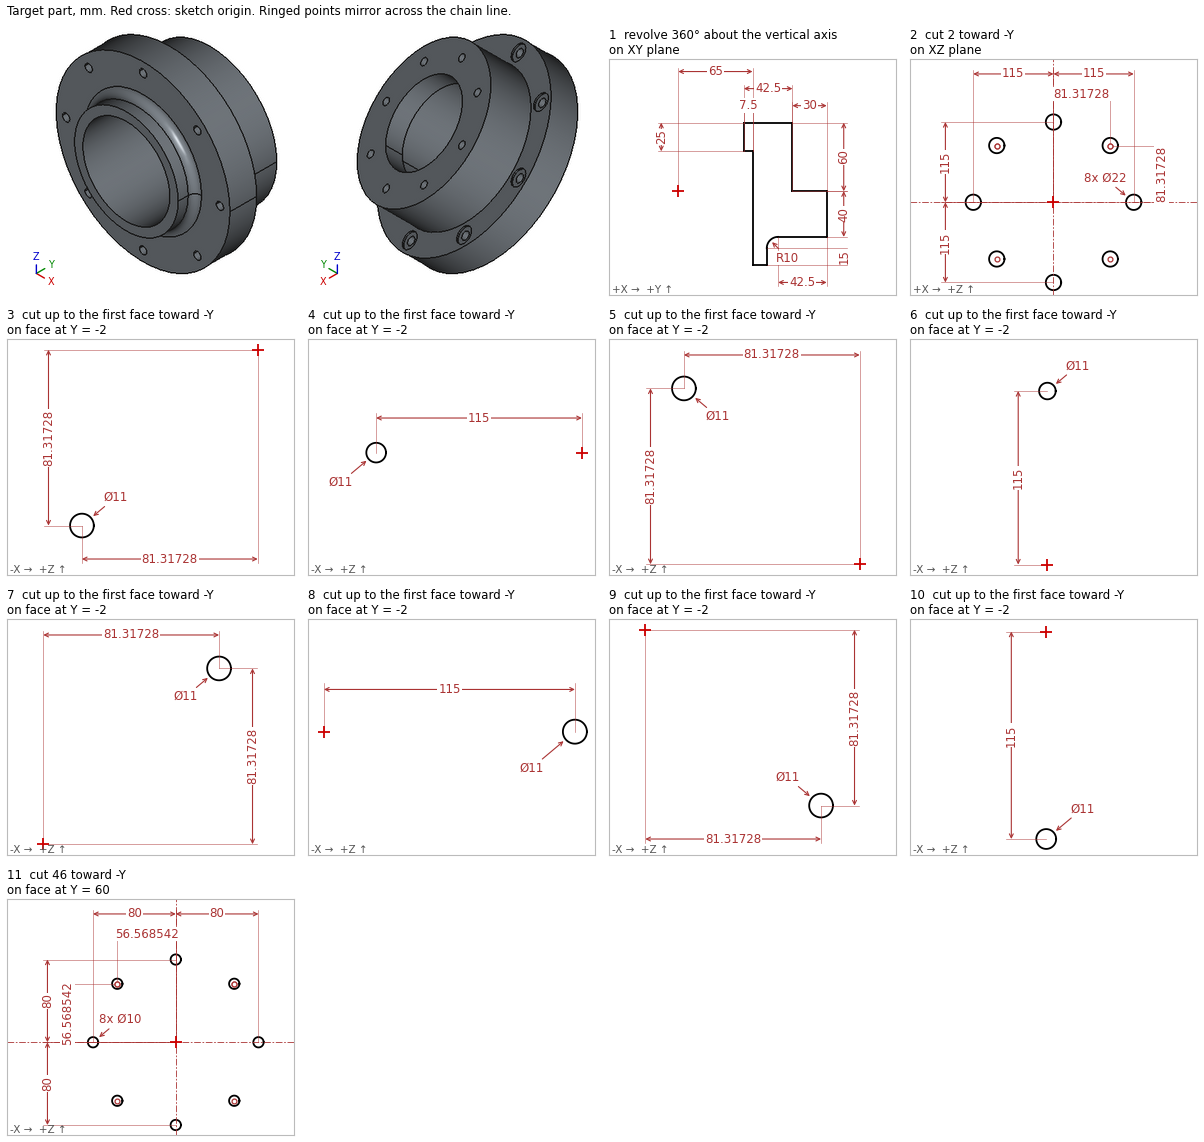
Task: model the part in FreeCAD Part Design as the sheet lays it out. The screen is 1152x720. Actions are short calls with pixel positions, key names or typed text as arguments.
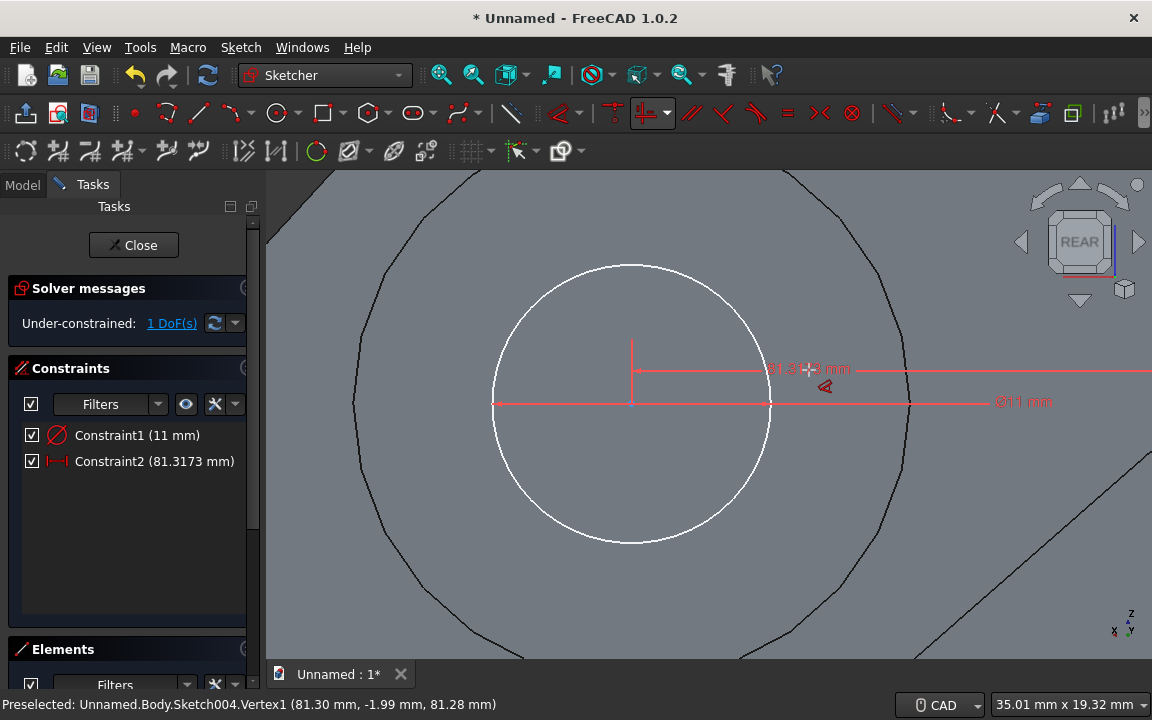
click(632, 404)
click(598, 518)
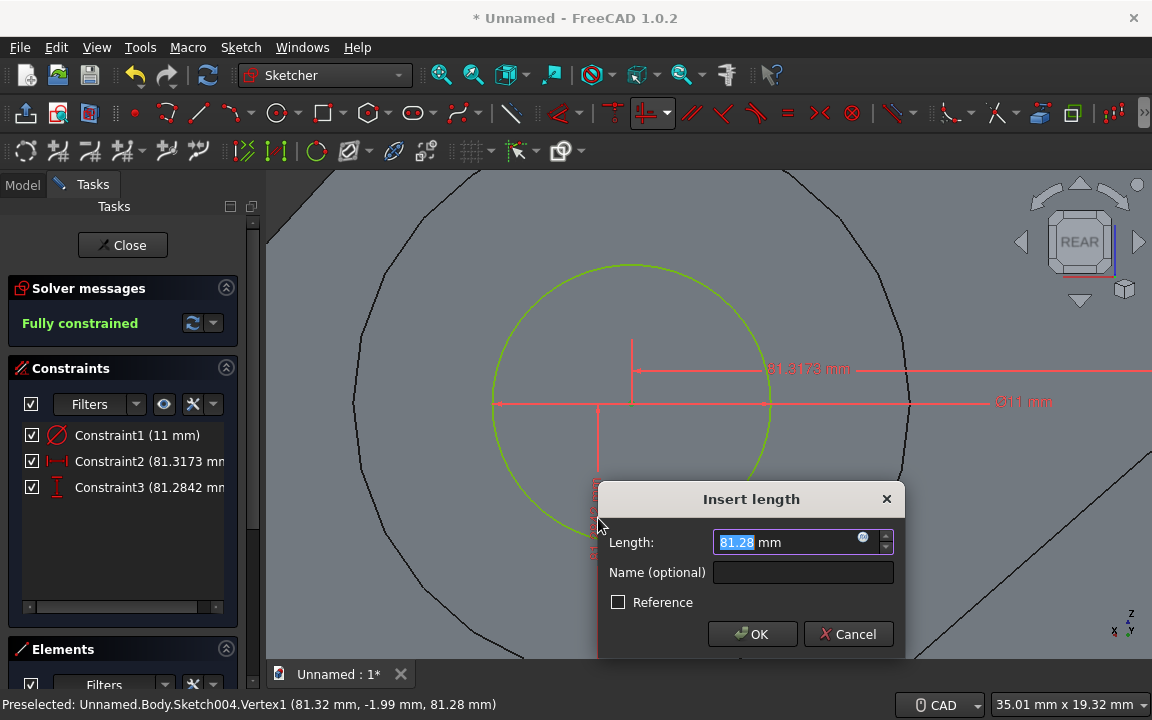
text(81.31728)
key(Return)
key(Escape)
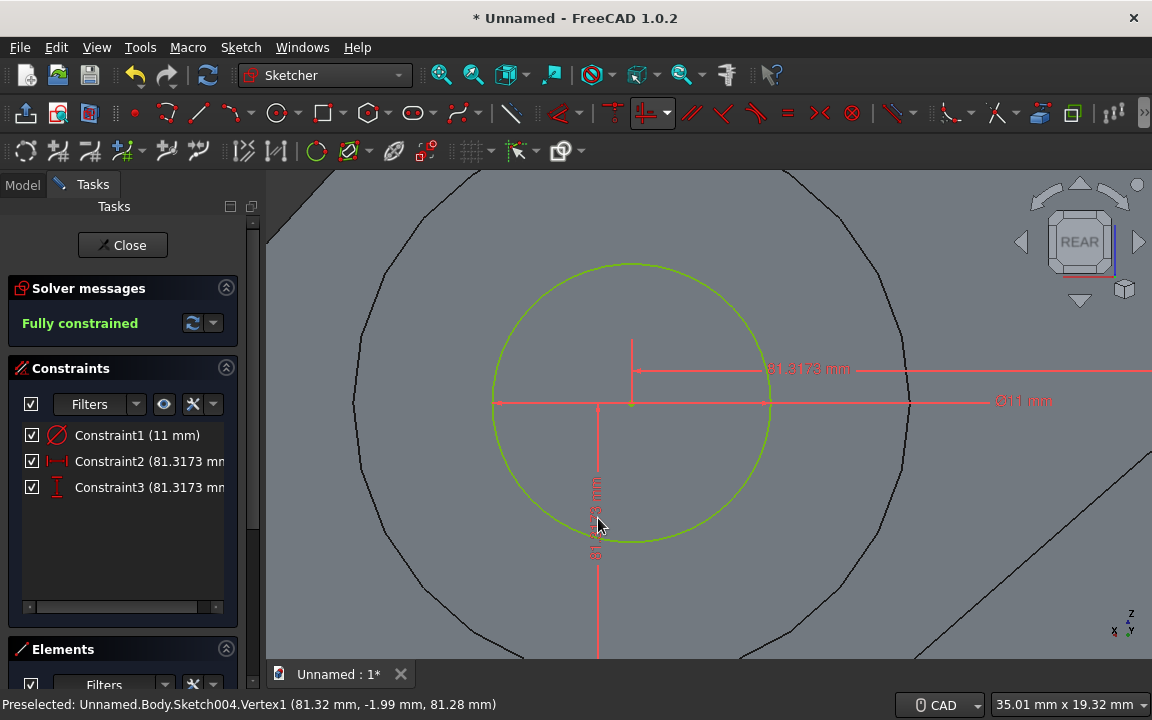
click(123, 245)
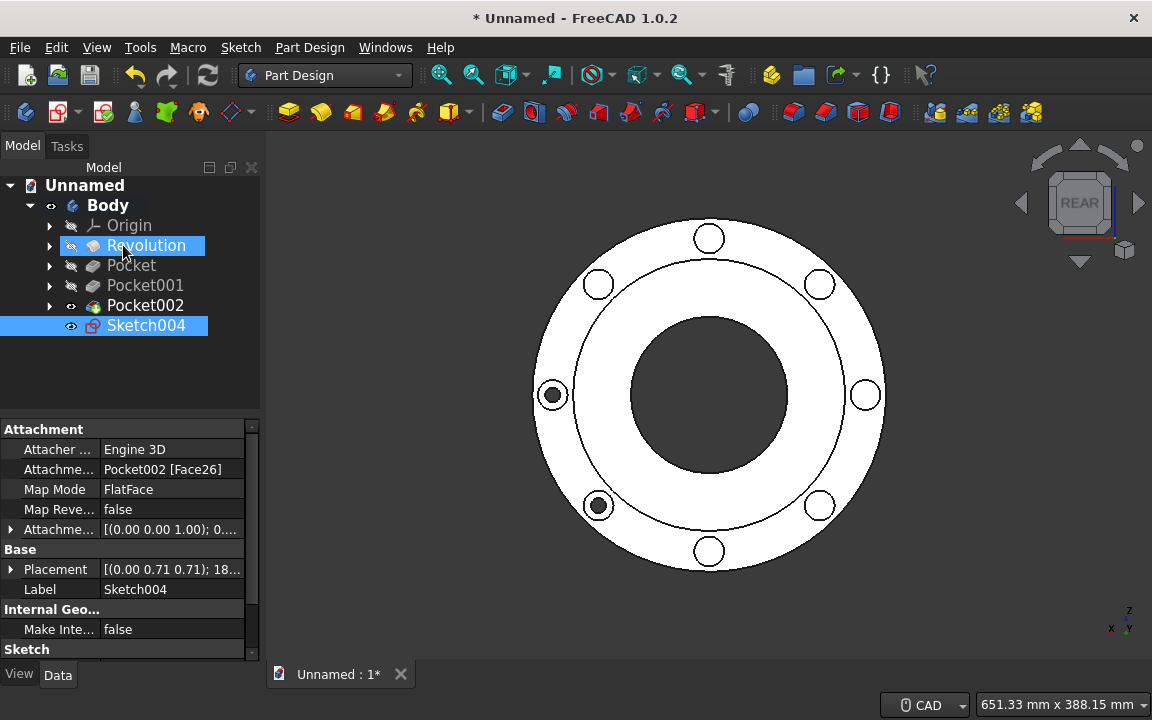
click(504, 112)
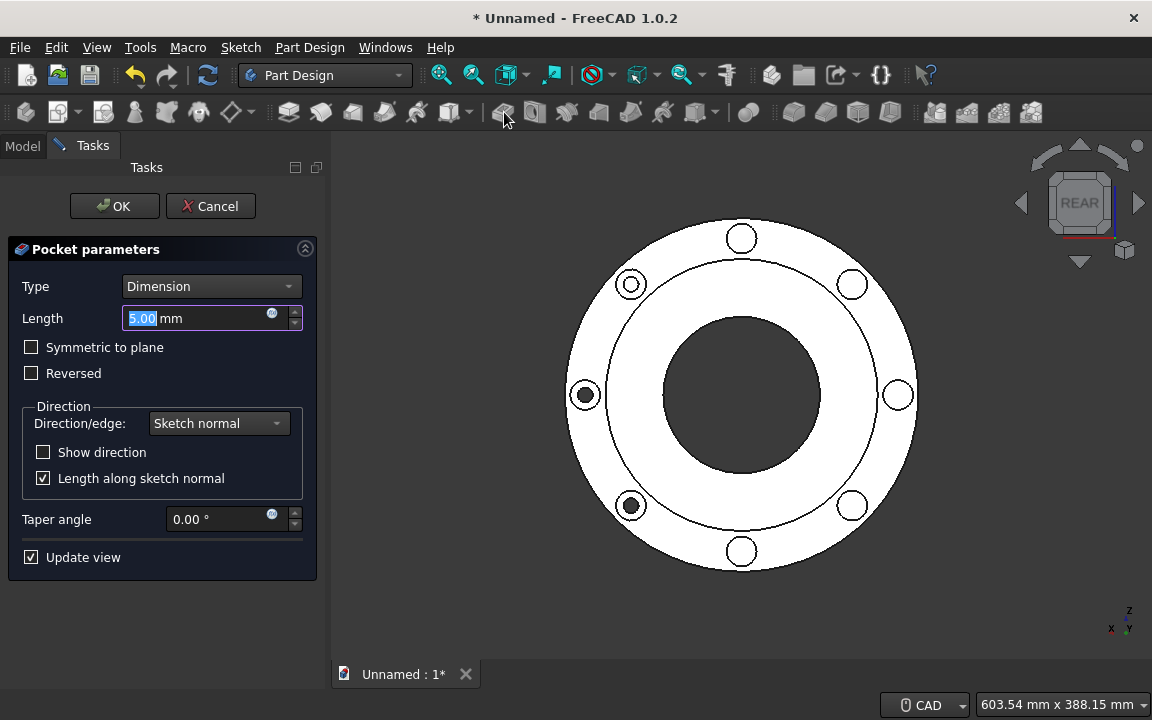
click(212, 286)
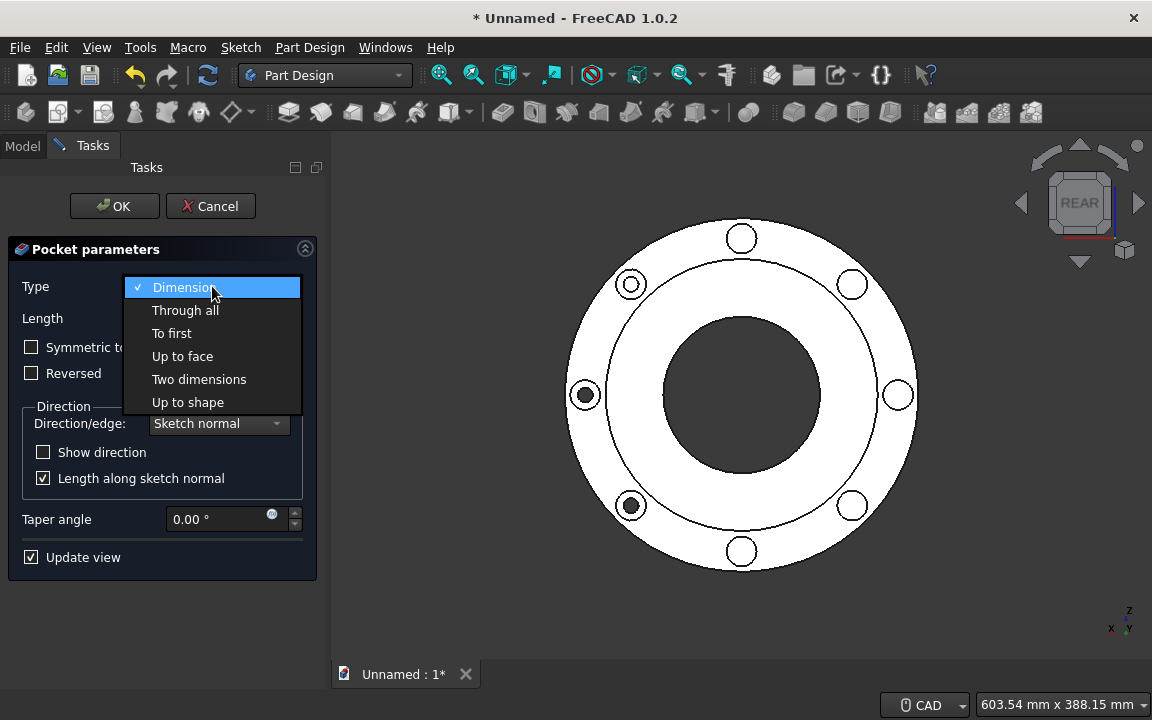
click(212, 334)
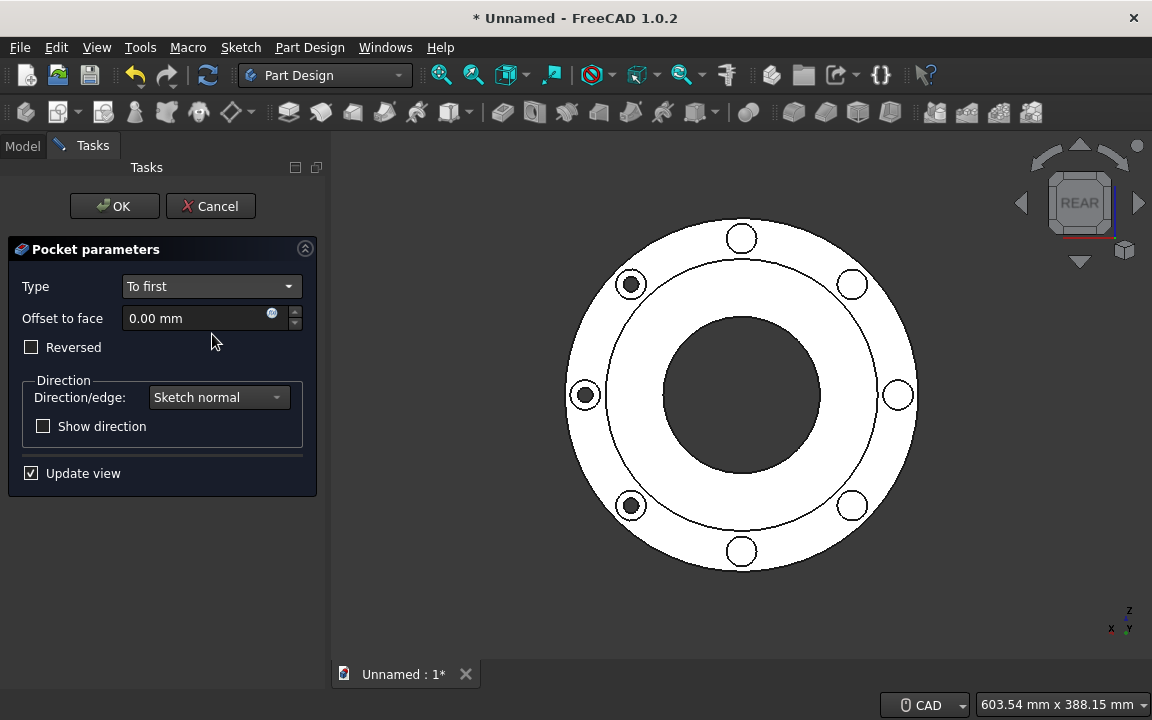
click(115, 206)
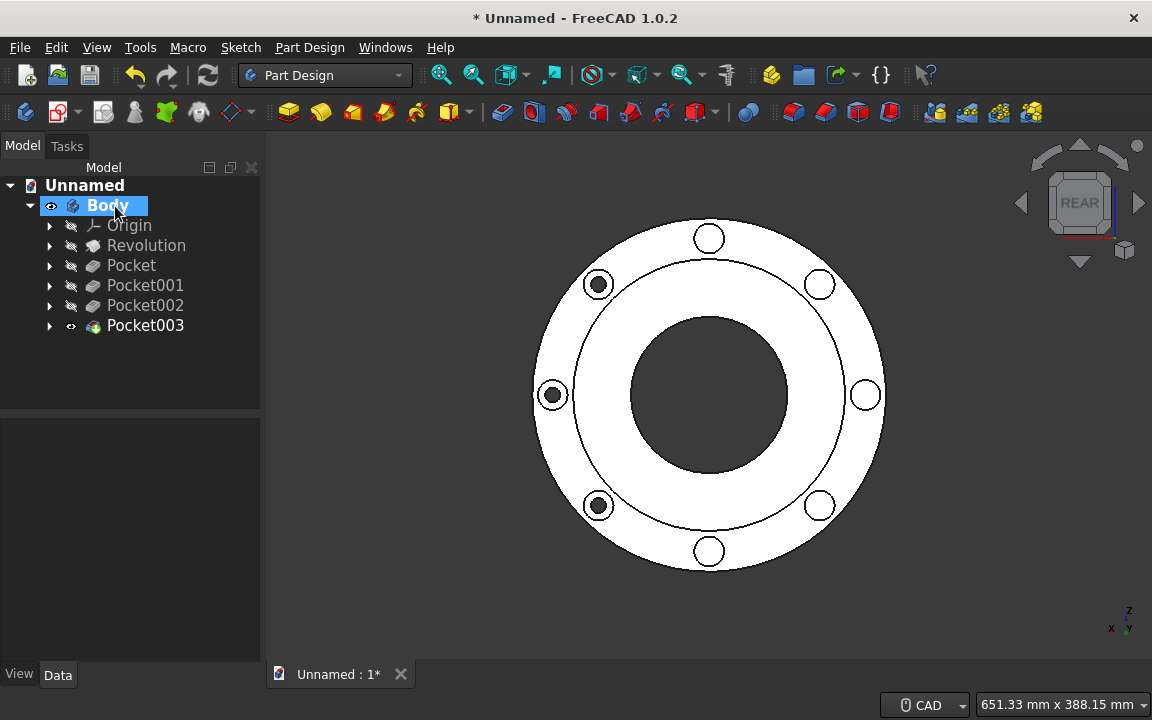
click(709, 238)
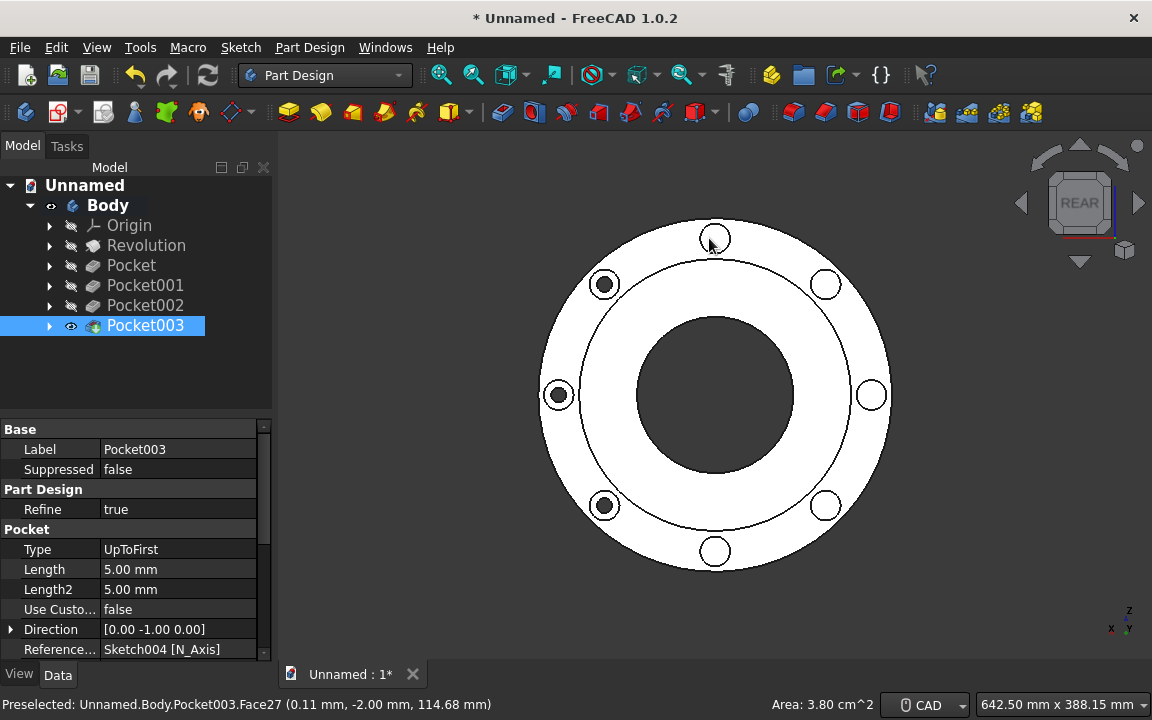
click(58, 112)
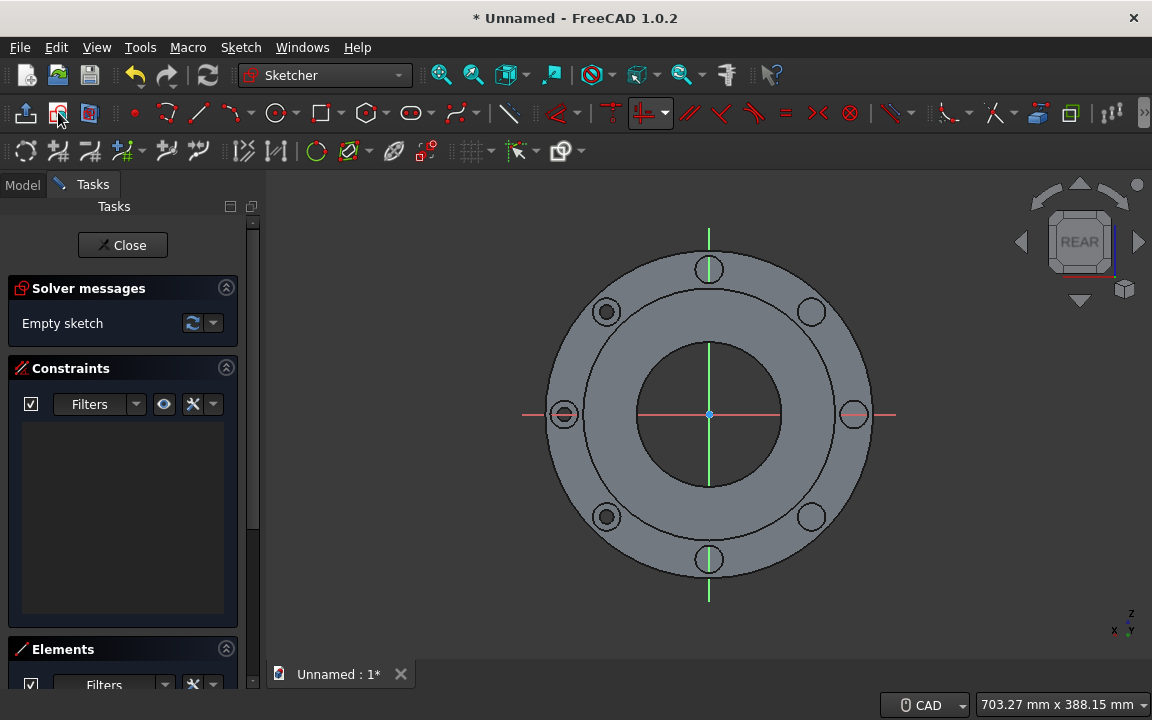
click(90, 114)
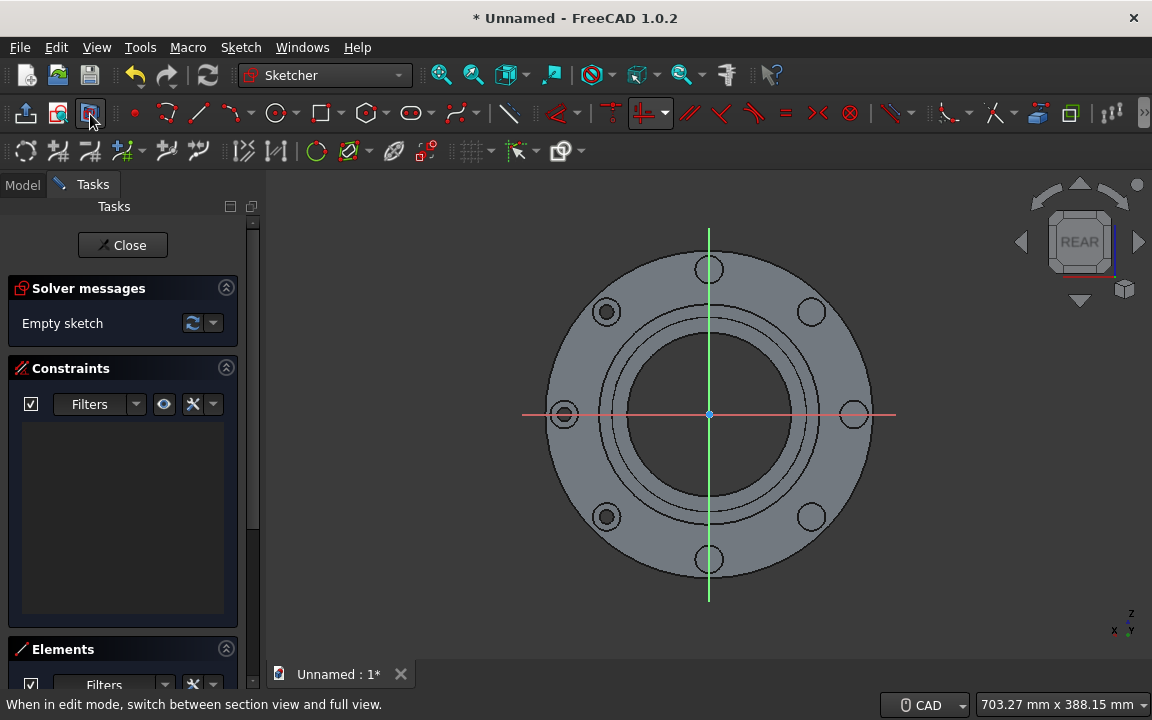
scroll(713, 262, up, 15)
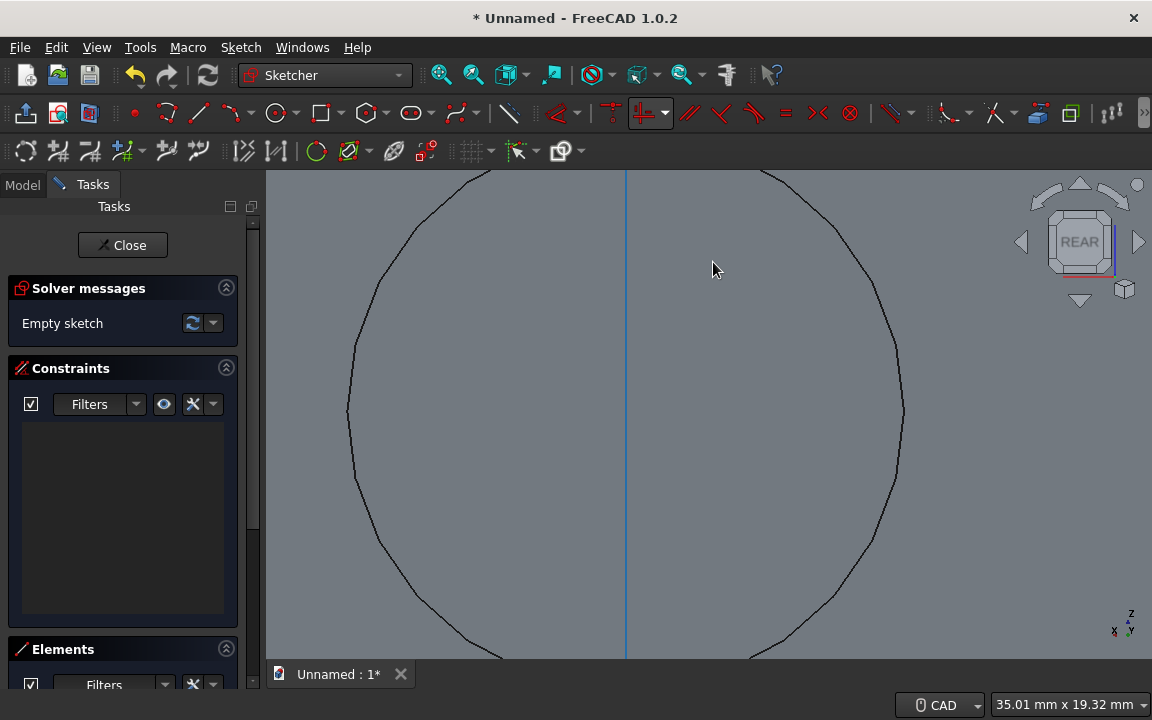
click(276, 114)